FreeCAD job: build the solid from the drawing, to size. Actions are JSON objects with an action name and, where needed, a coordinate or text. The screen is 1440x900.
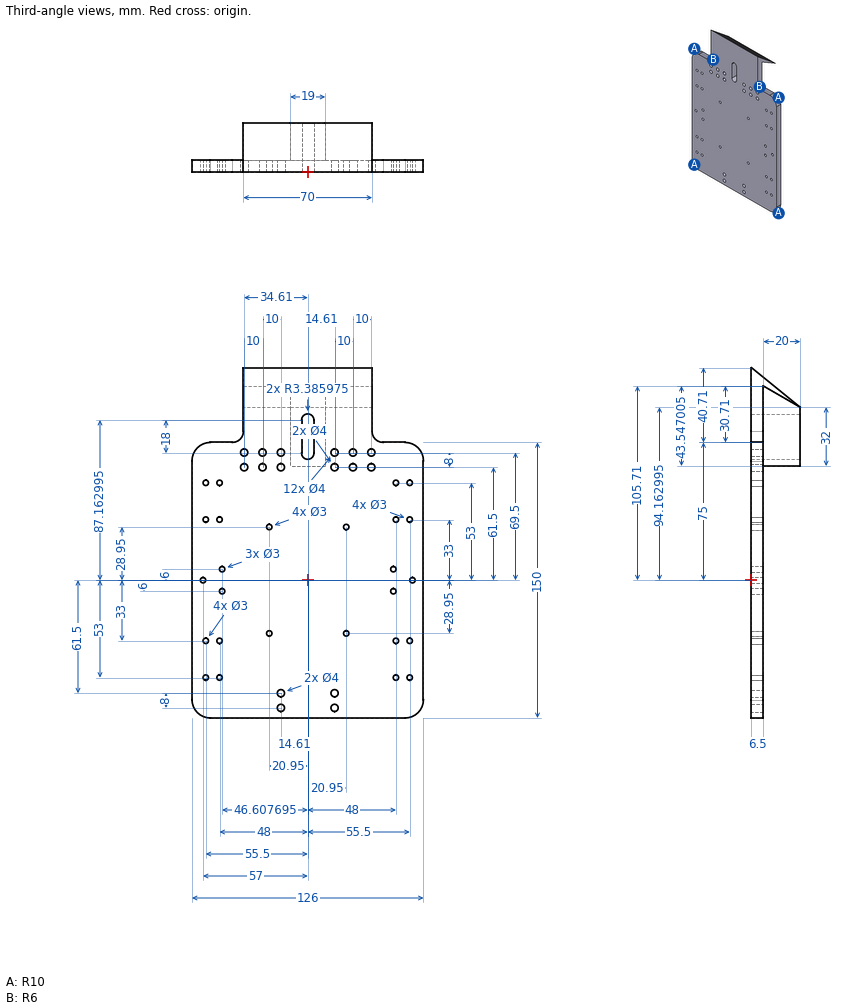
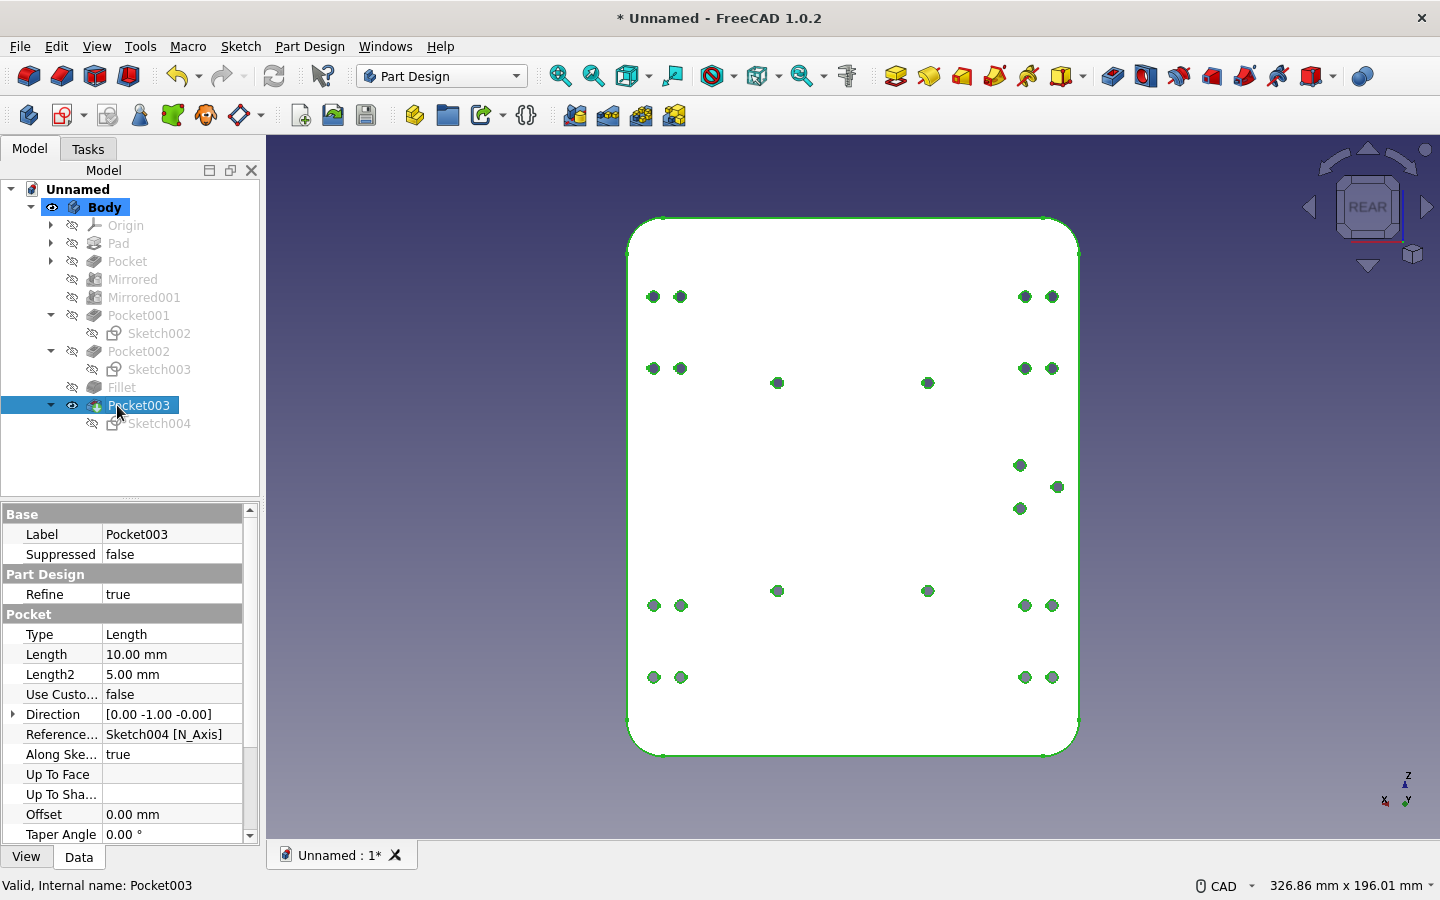
{"action": "left_click", "coordinate": [575, 116]}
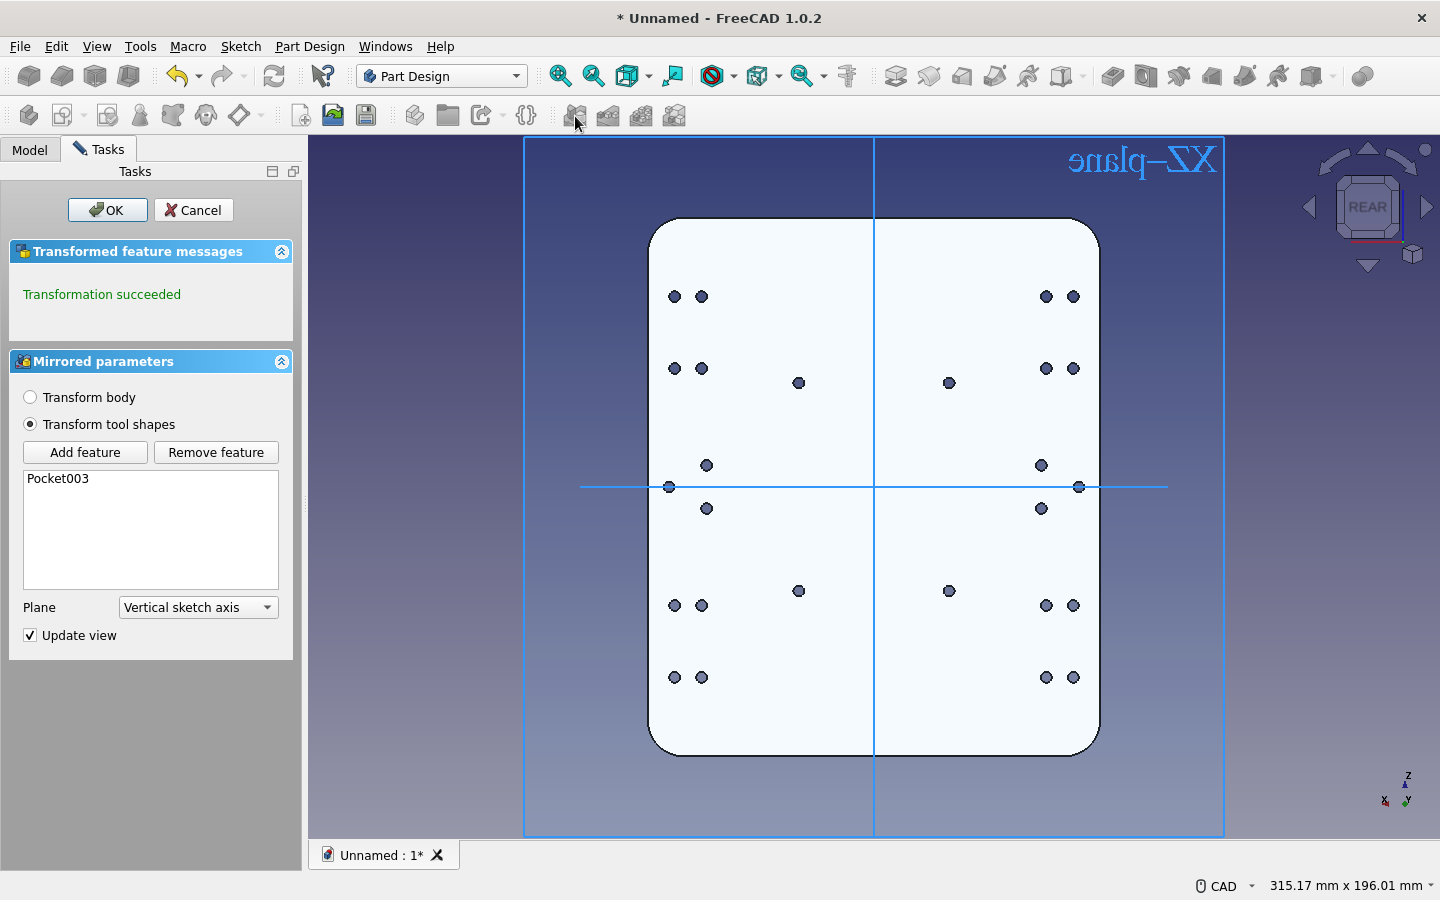
{"action": "left_click", "coordinate": [199, 608]}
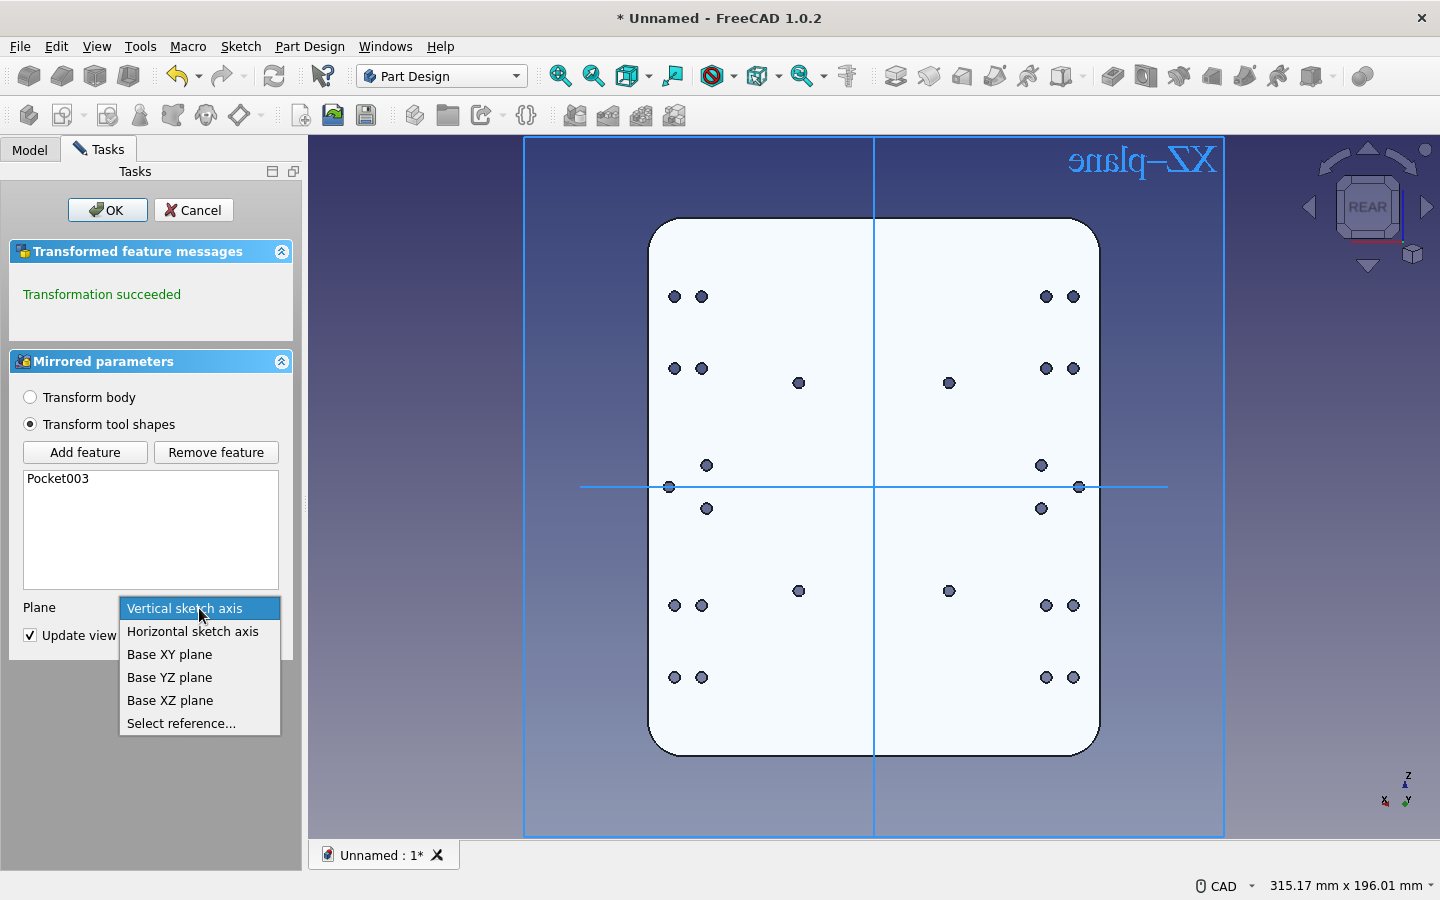
{"action": "left_click", "coordinate": [198, 678]}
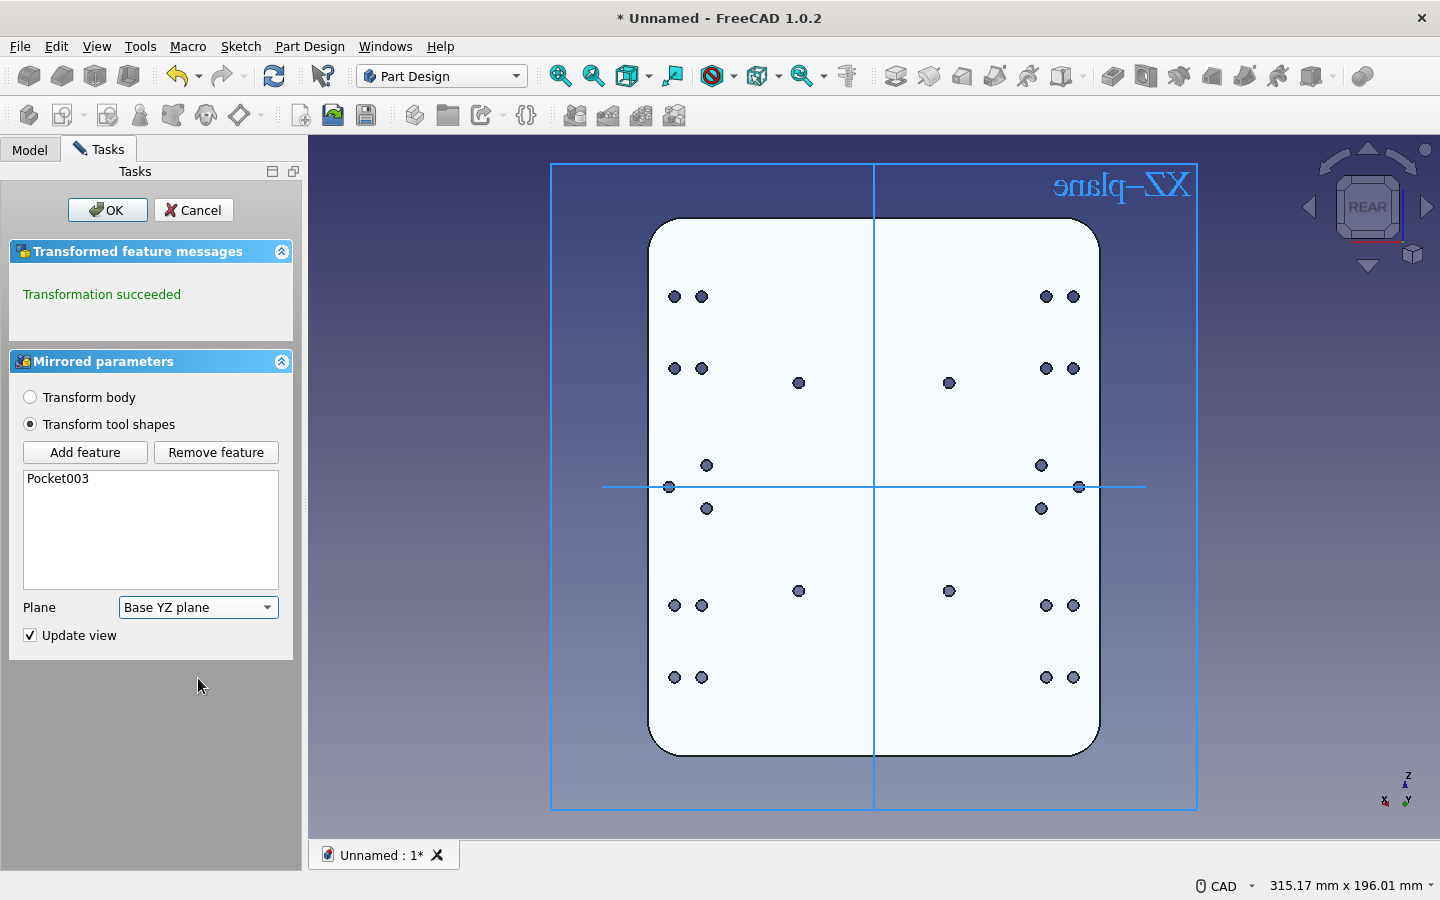
{"action": "left_click", "coordinate": [108, 210]}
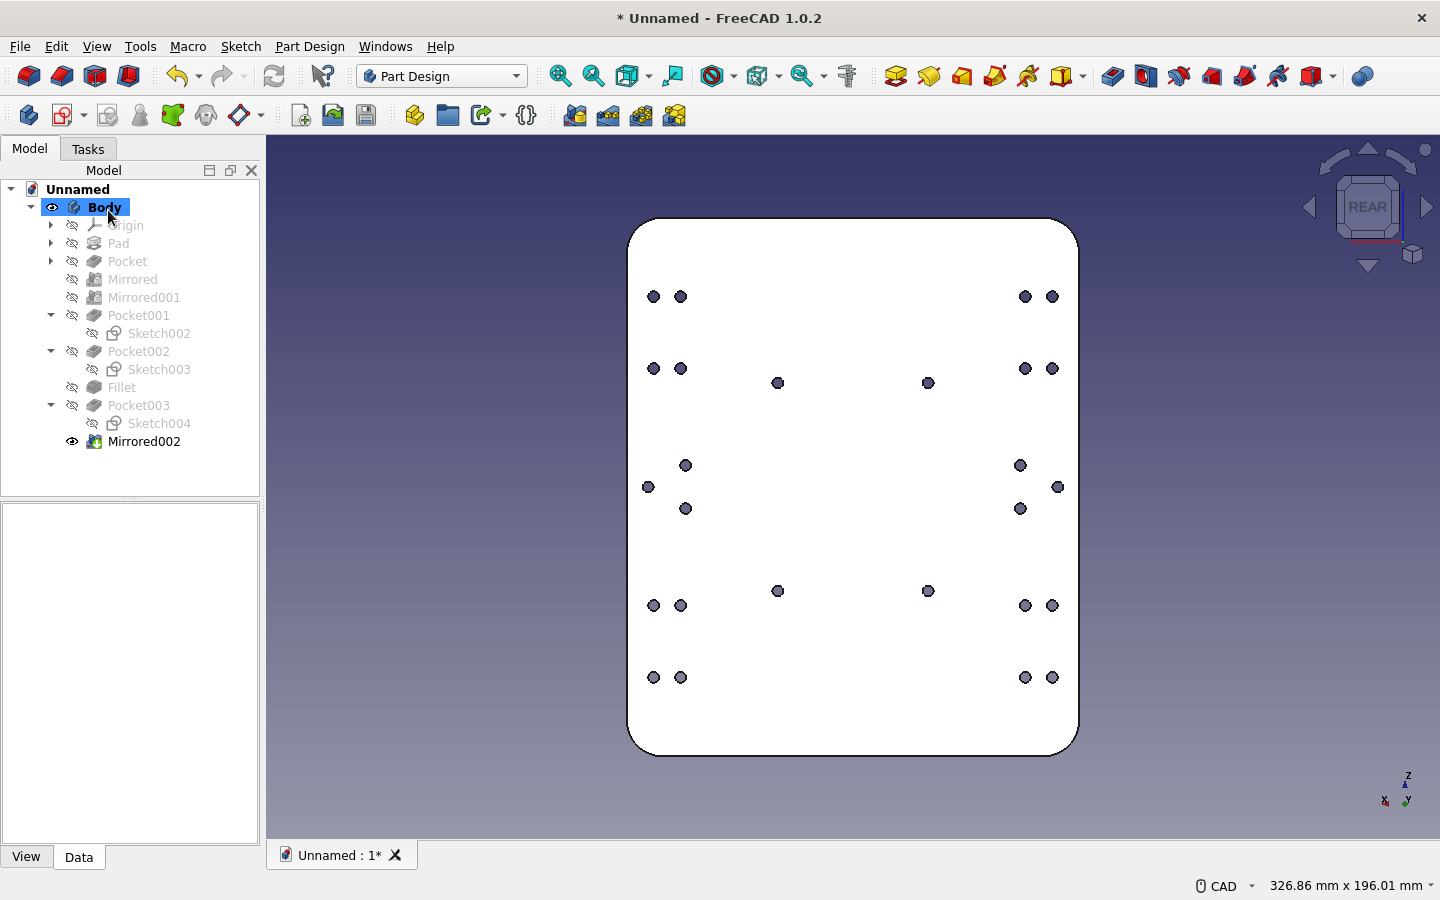
{"action": "left_click", "coordinate": [853, 486]}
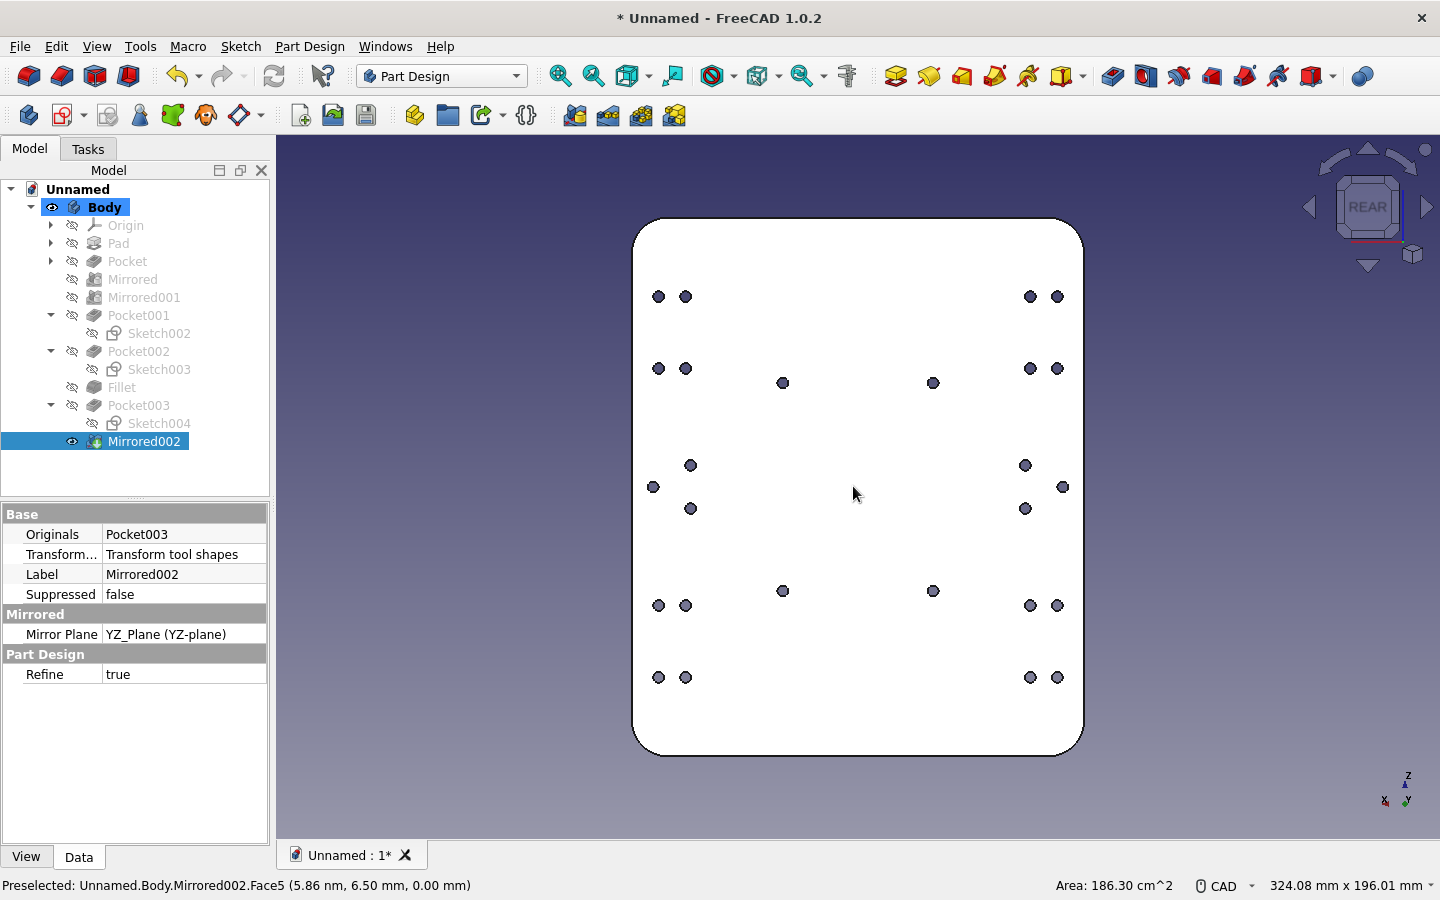
{"action": "left_click", "coordinate": [62, 116]}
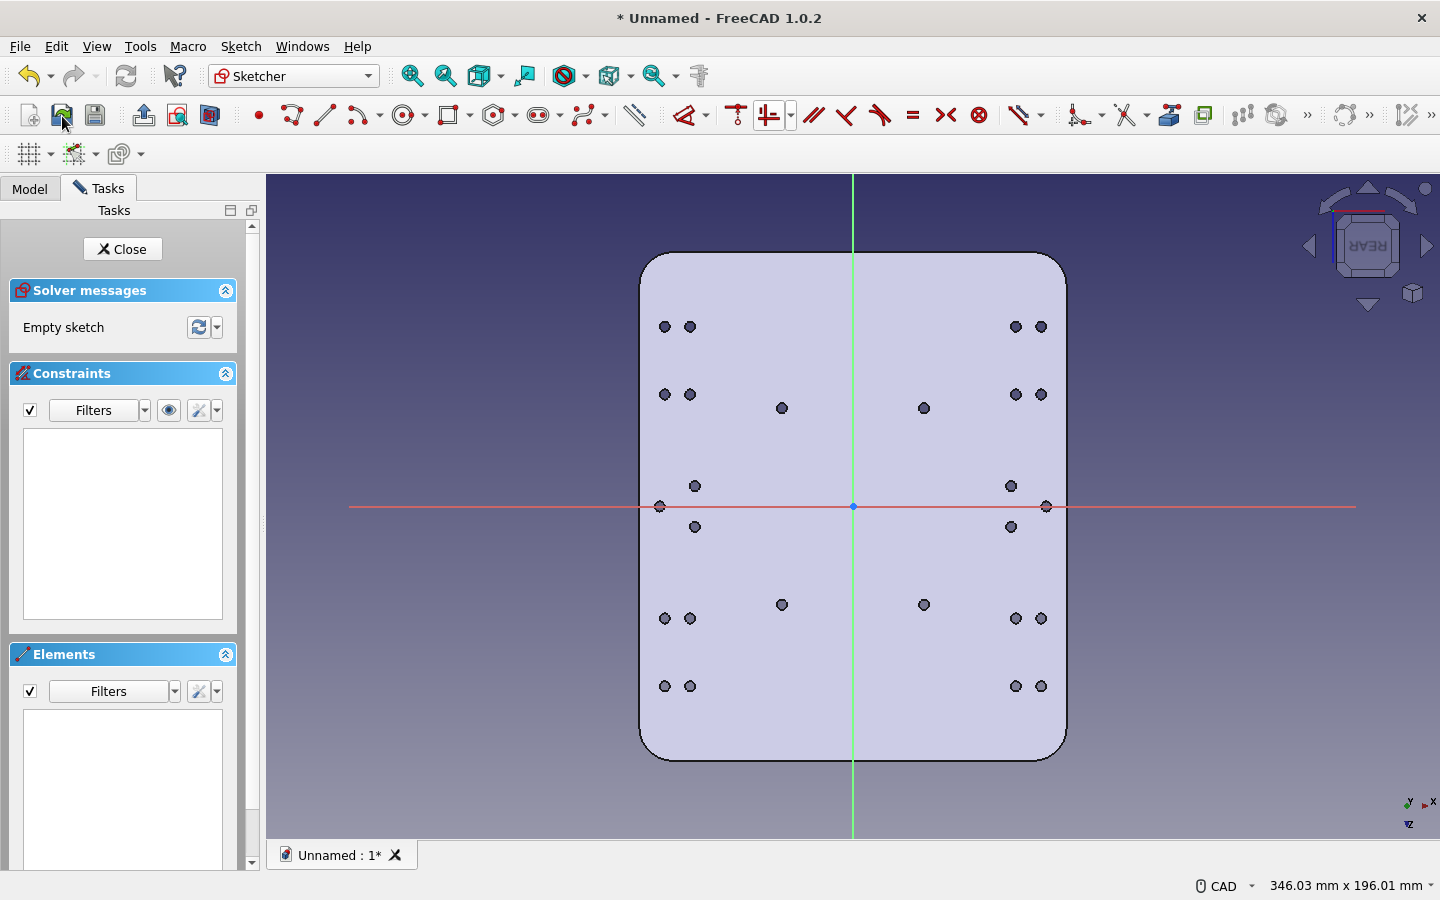
{"action": "scroll", "coordinate": [914, 751], "scroll_direction": "up", "scroll_amount": 12}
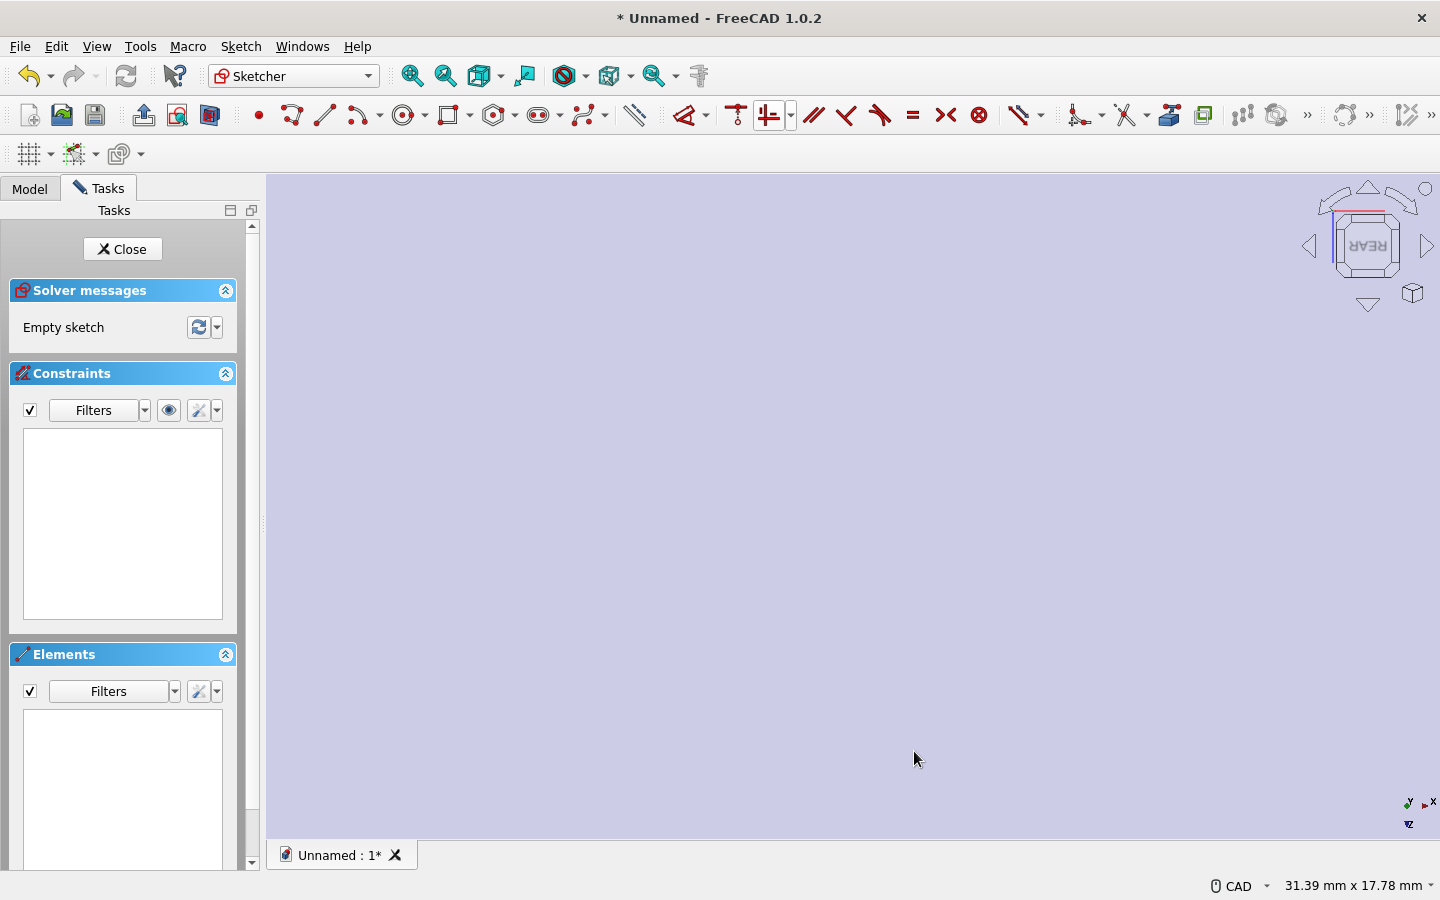
{"action": "left_click", "coordinate": [402, 116]}